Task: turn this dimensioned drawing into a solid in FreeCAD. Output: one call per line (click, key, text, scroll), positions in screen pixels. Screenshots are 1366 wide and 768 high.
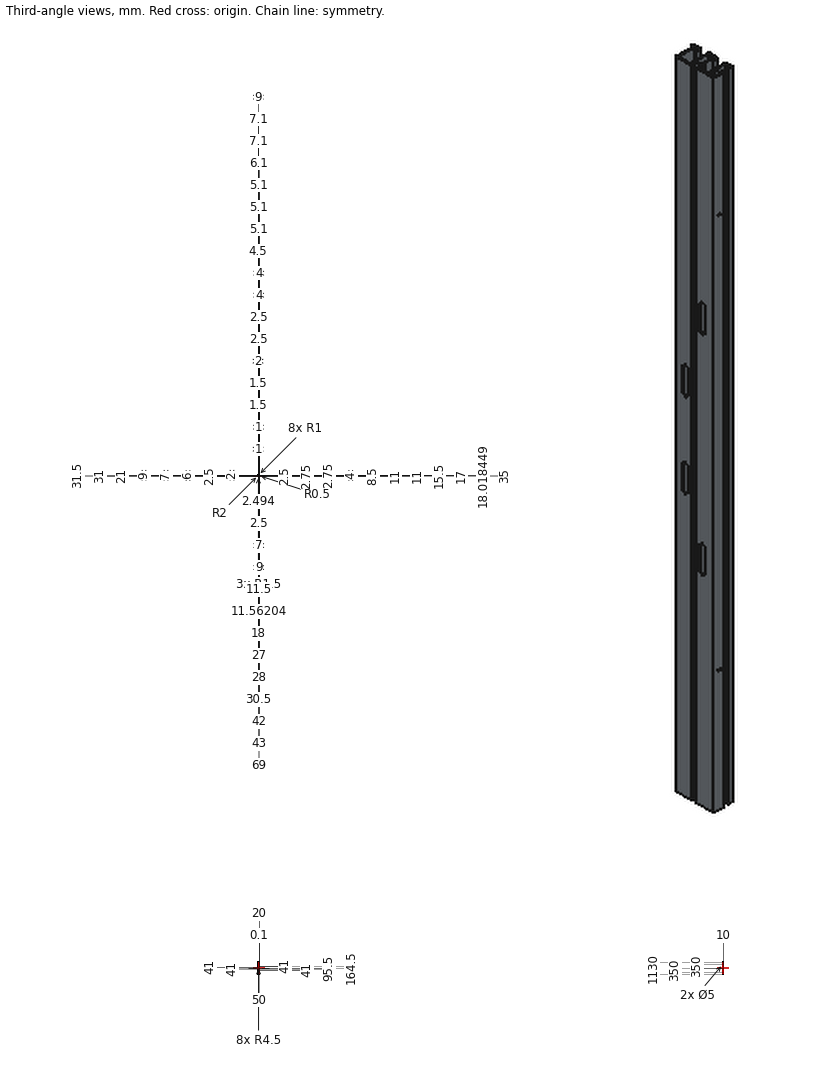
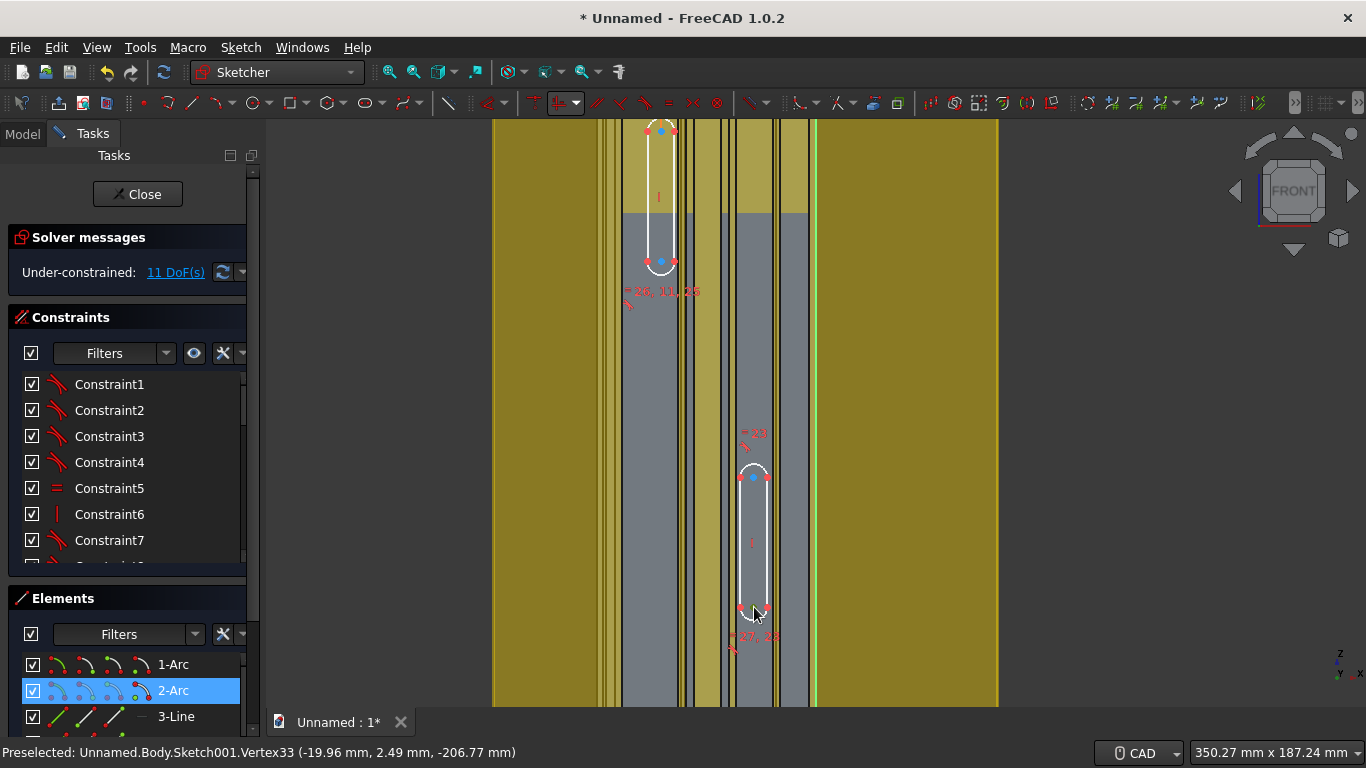
scroll(755, 609, down, 6)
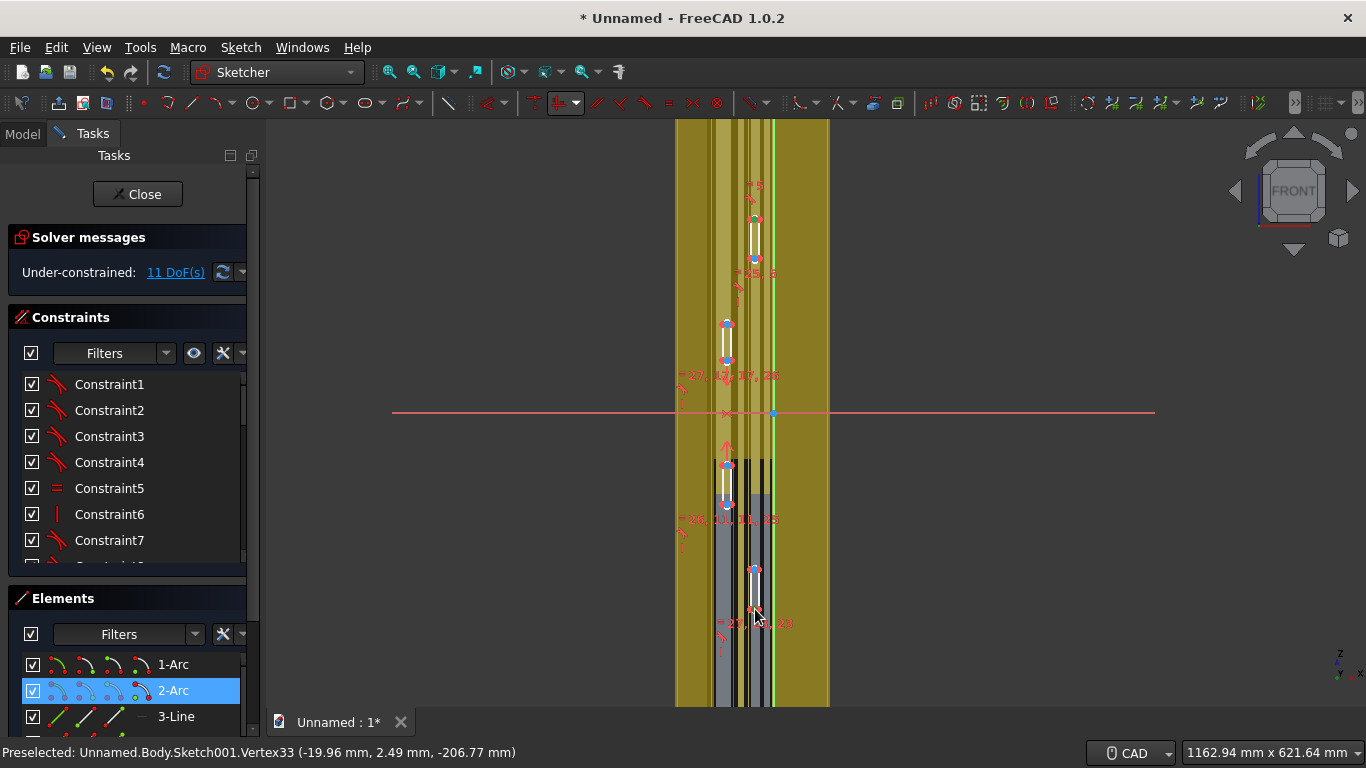
click(424, 413)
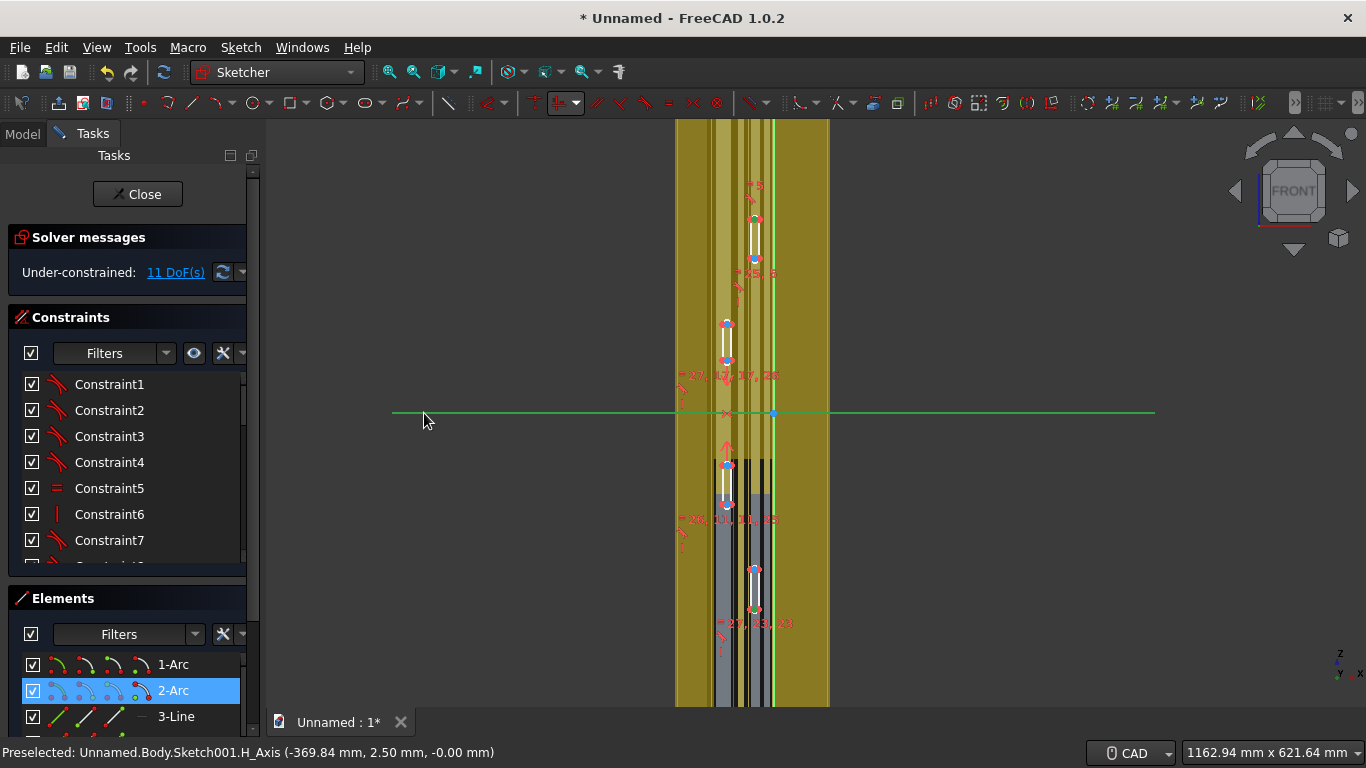
click(694, 104)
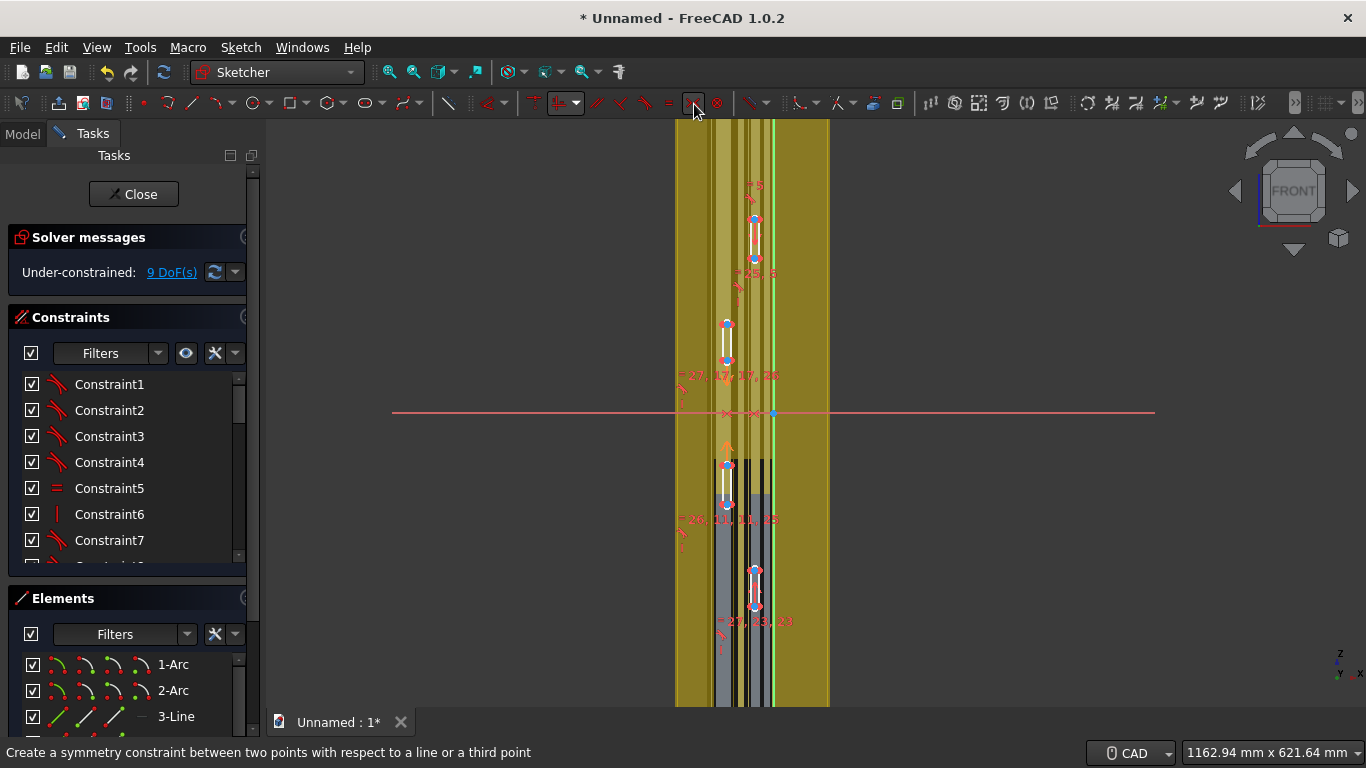
click(488, 104)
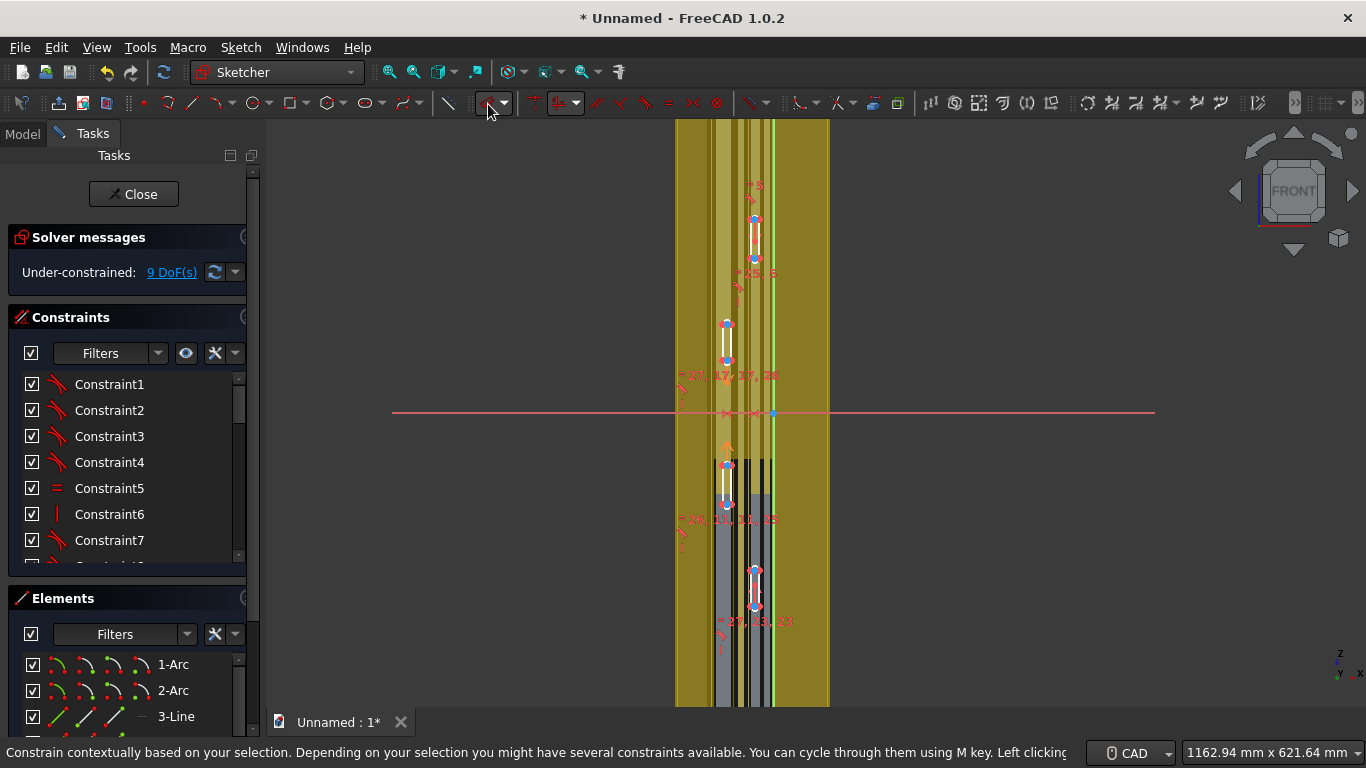
scroll(755, 263, up, 12)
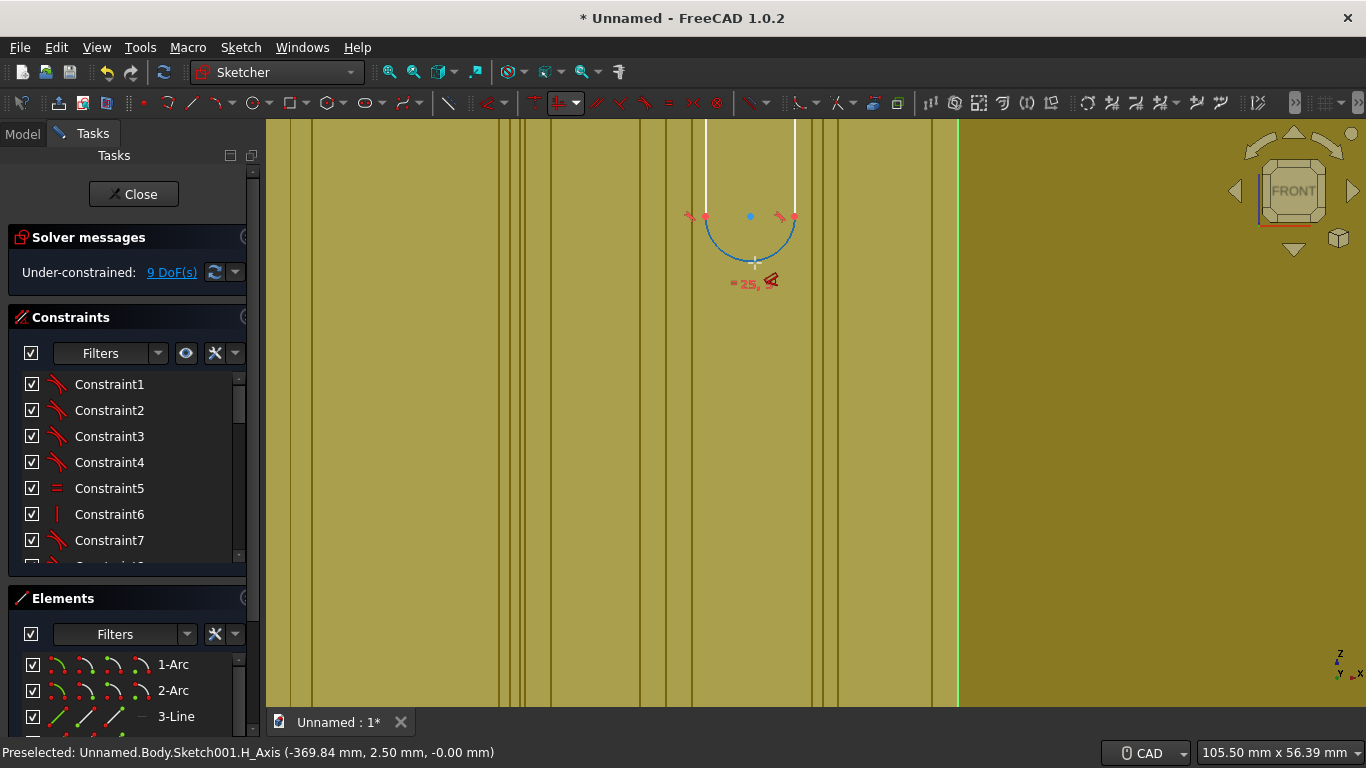
click(750, 261)
click(750, 293)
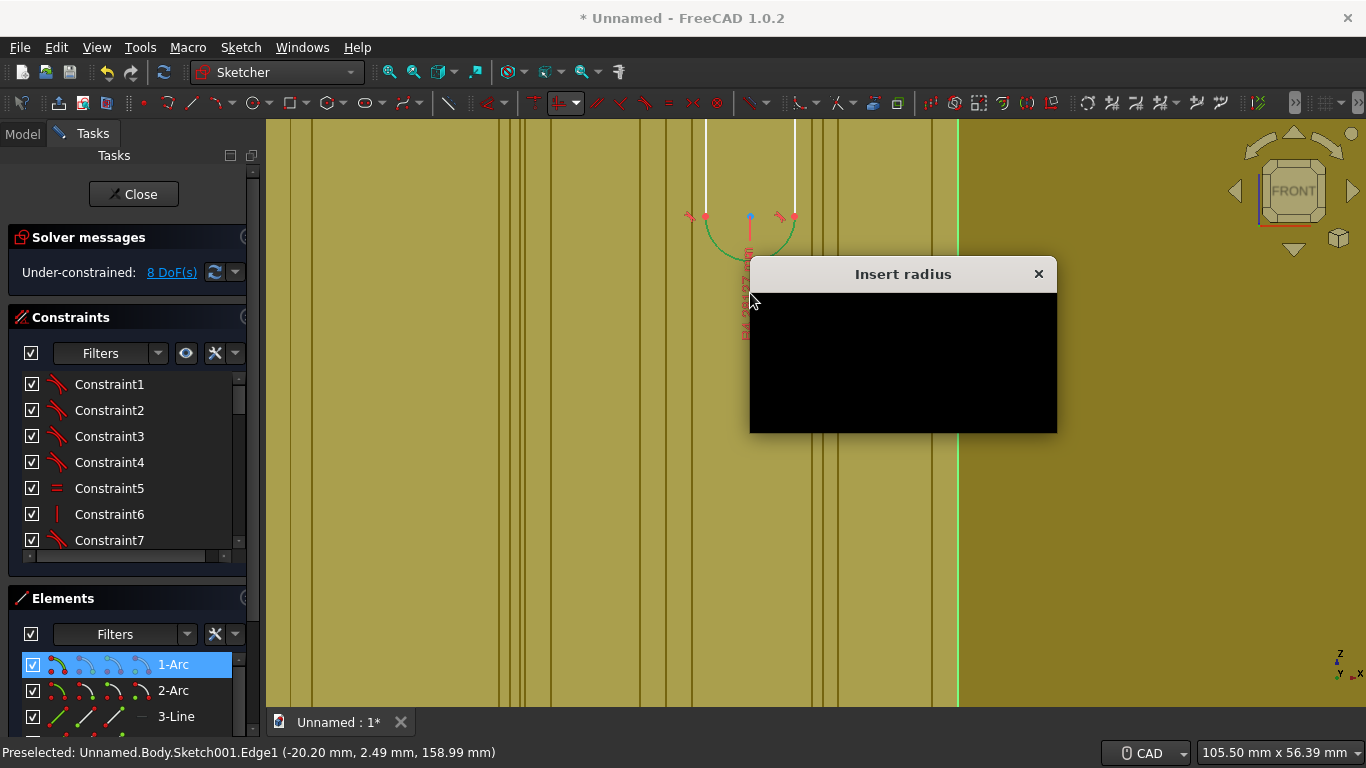
text(4.5)
key(Return)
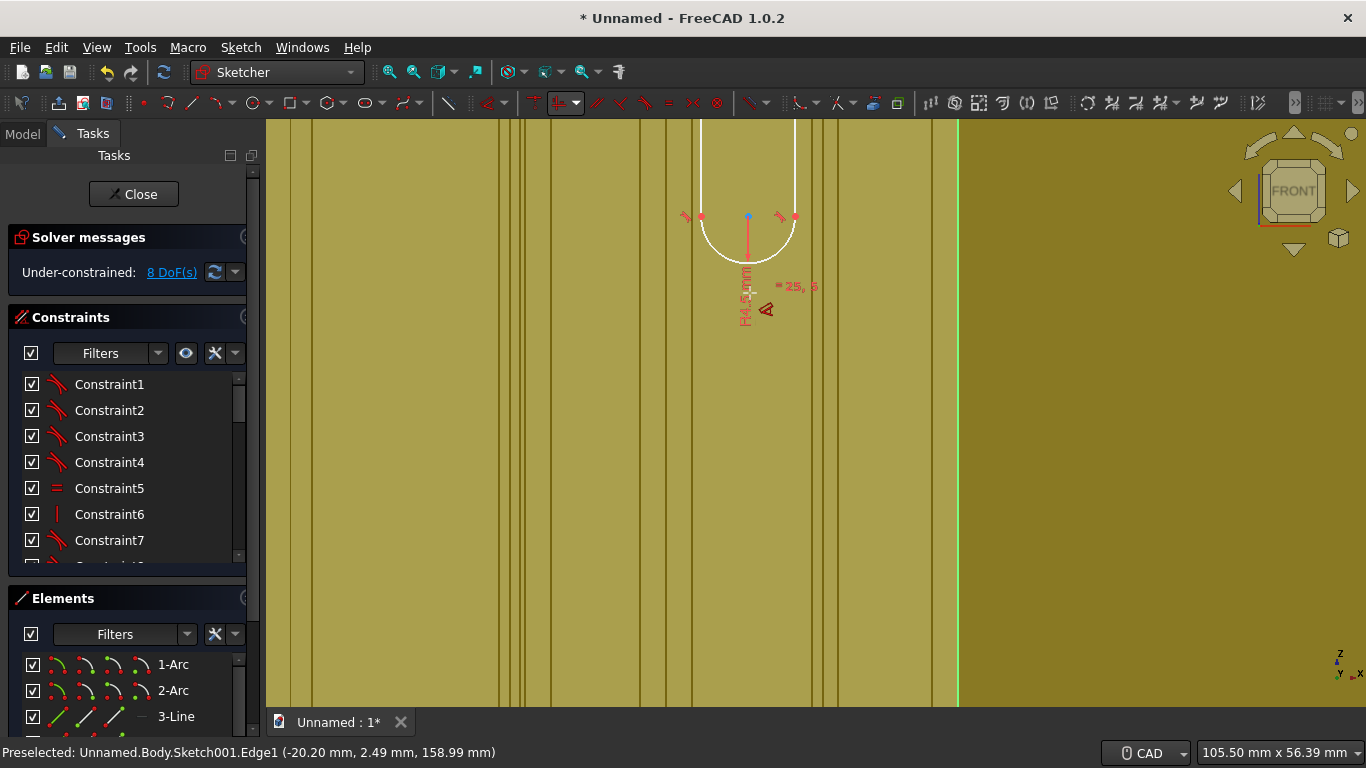
scroll(755, 263, down, 12)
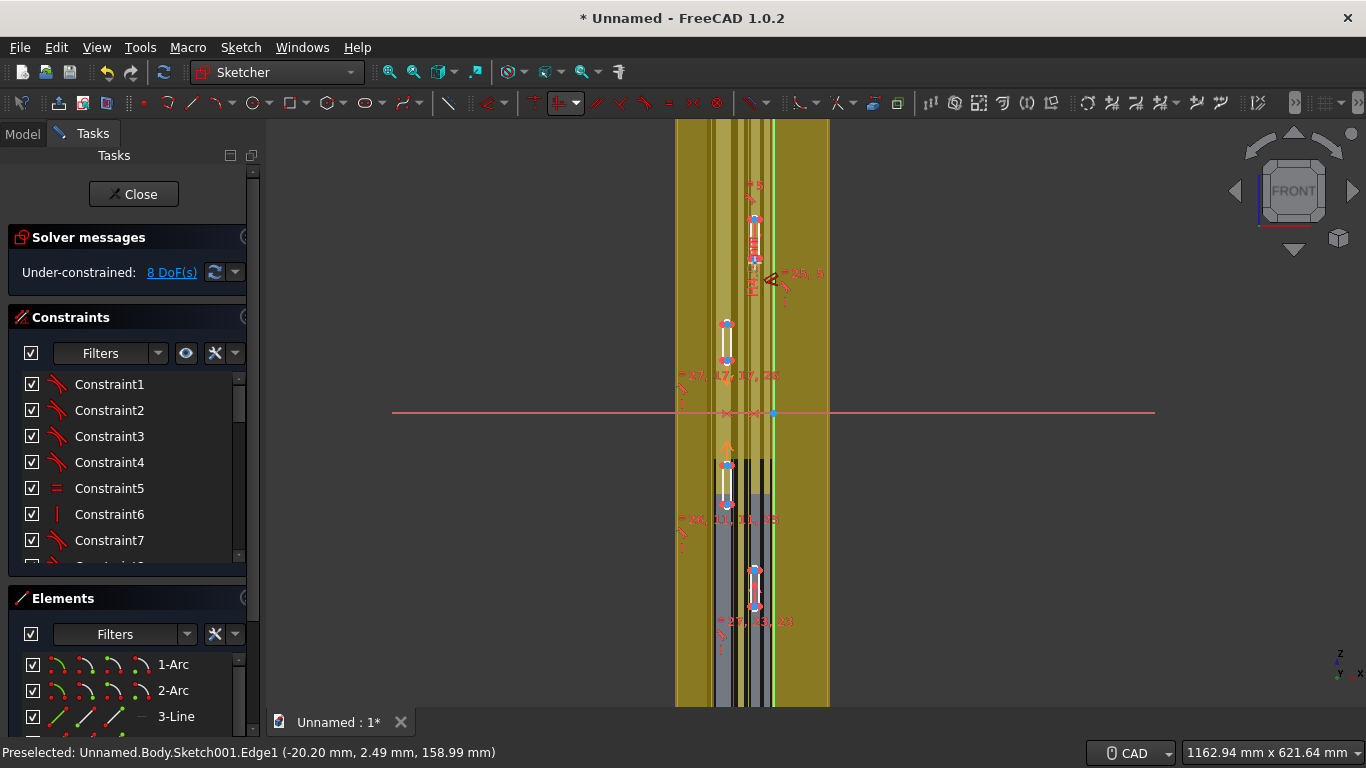
scroll(751, 247, up, 3)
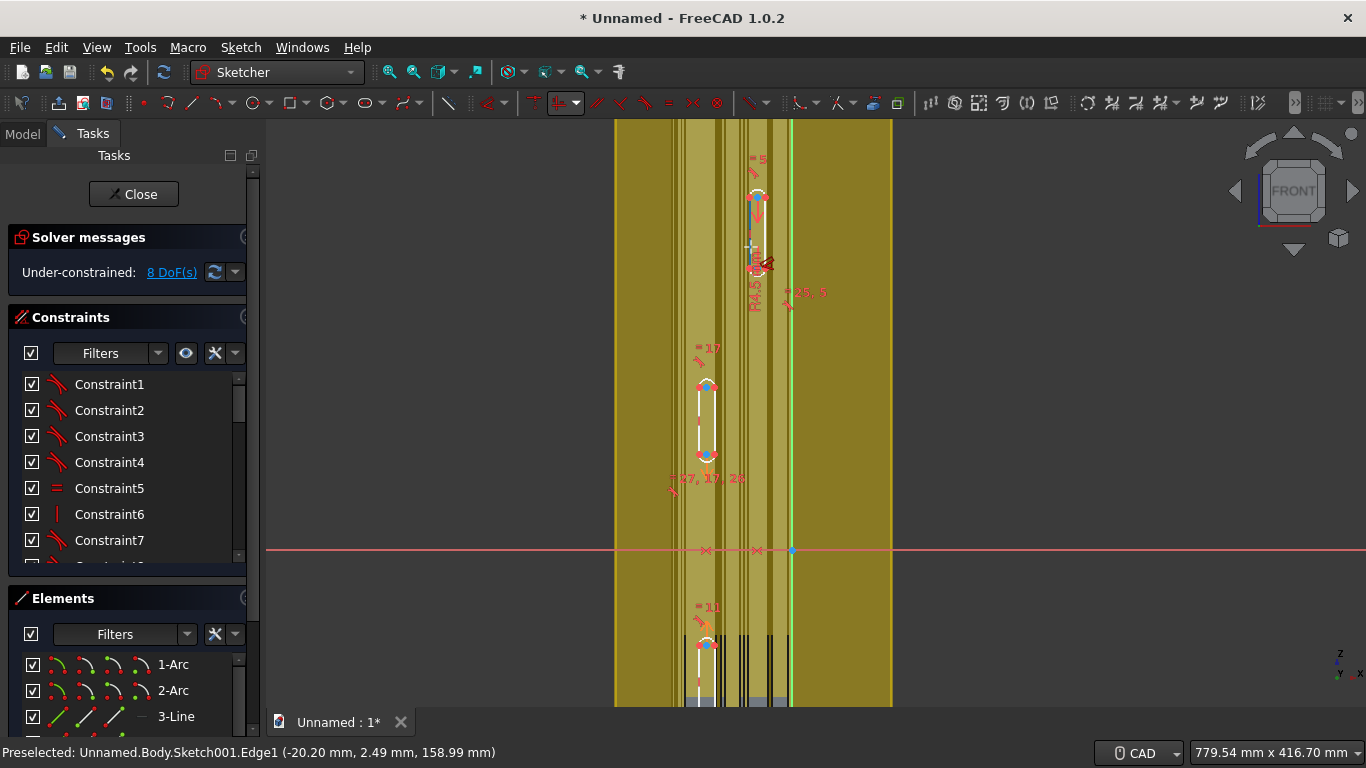
click(750, 247)
click(716, 233)